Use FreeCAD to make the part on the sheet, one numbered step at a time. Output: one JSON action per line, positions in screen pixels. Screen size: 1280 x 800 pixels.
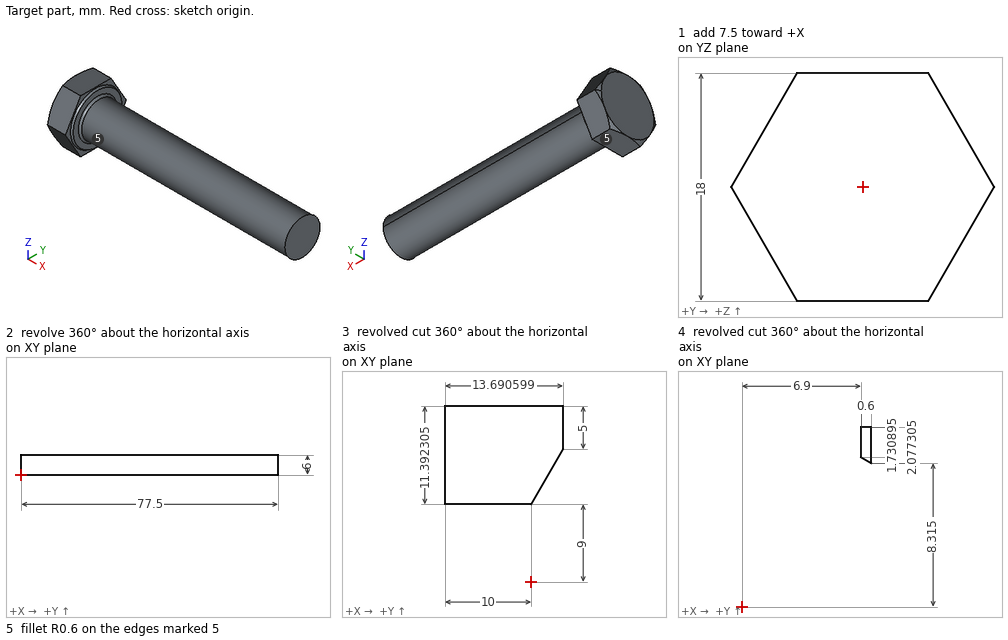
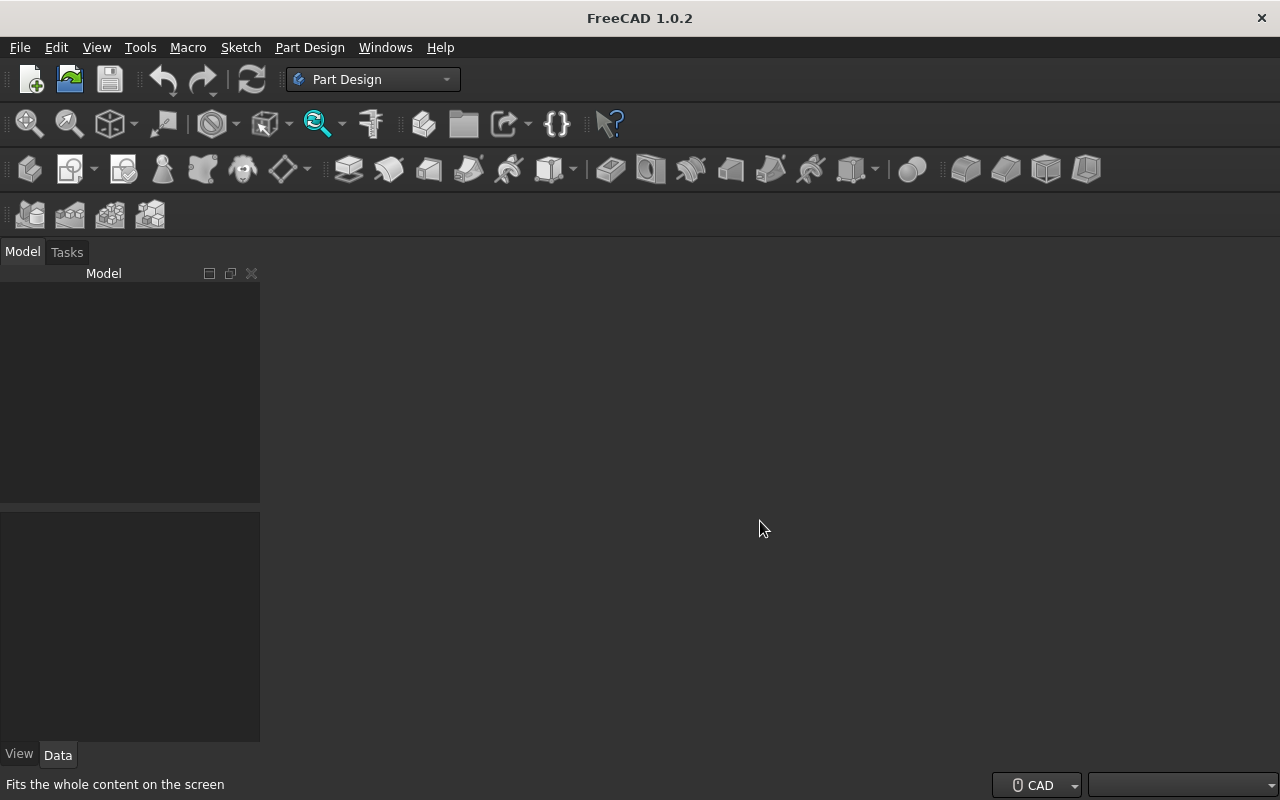
{"action": "left_click", "coordinate": [30, 80]}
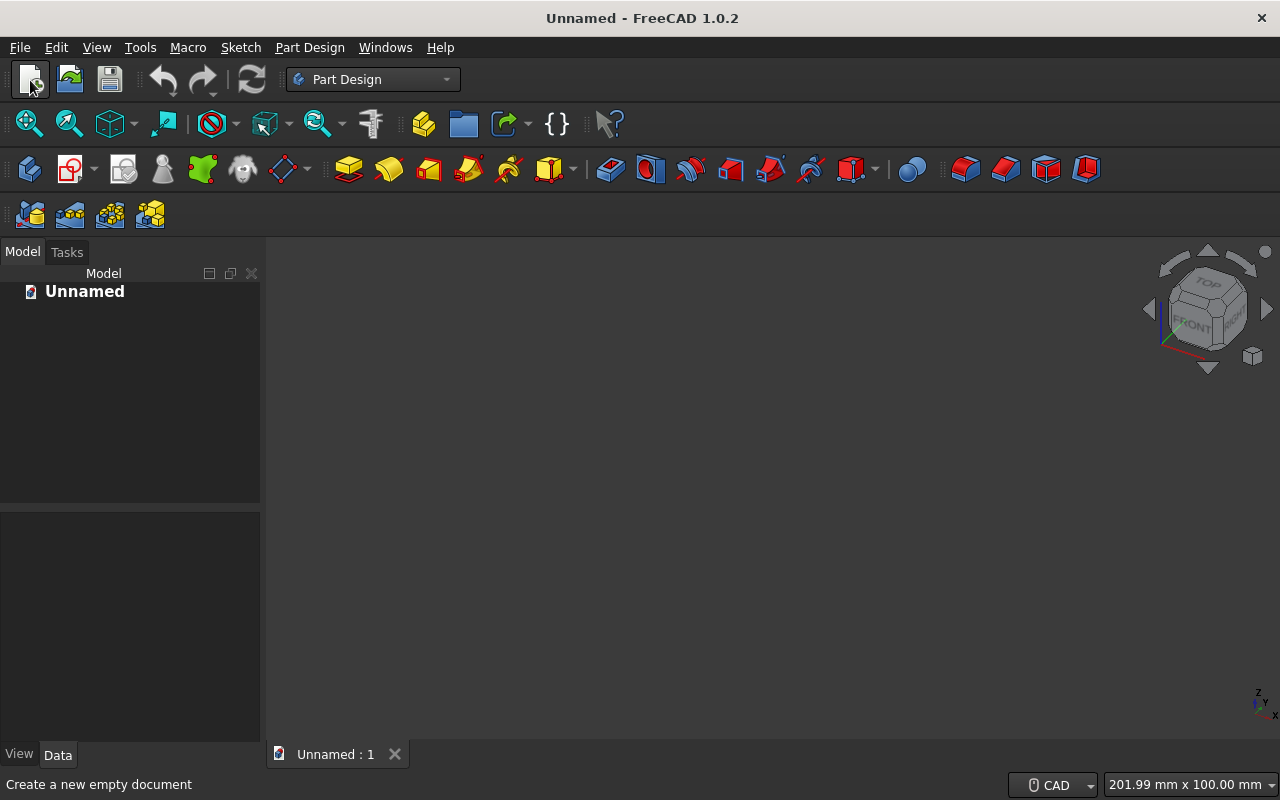
{"action": "left_click", "coordinate": [70, 170]}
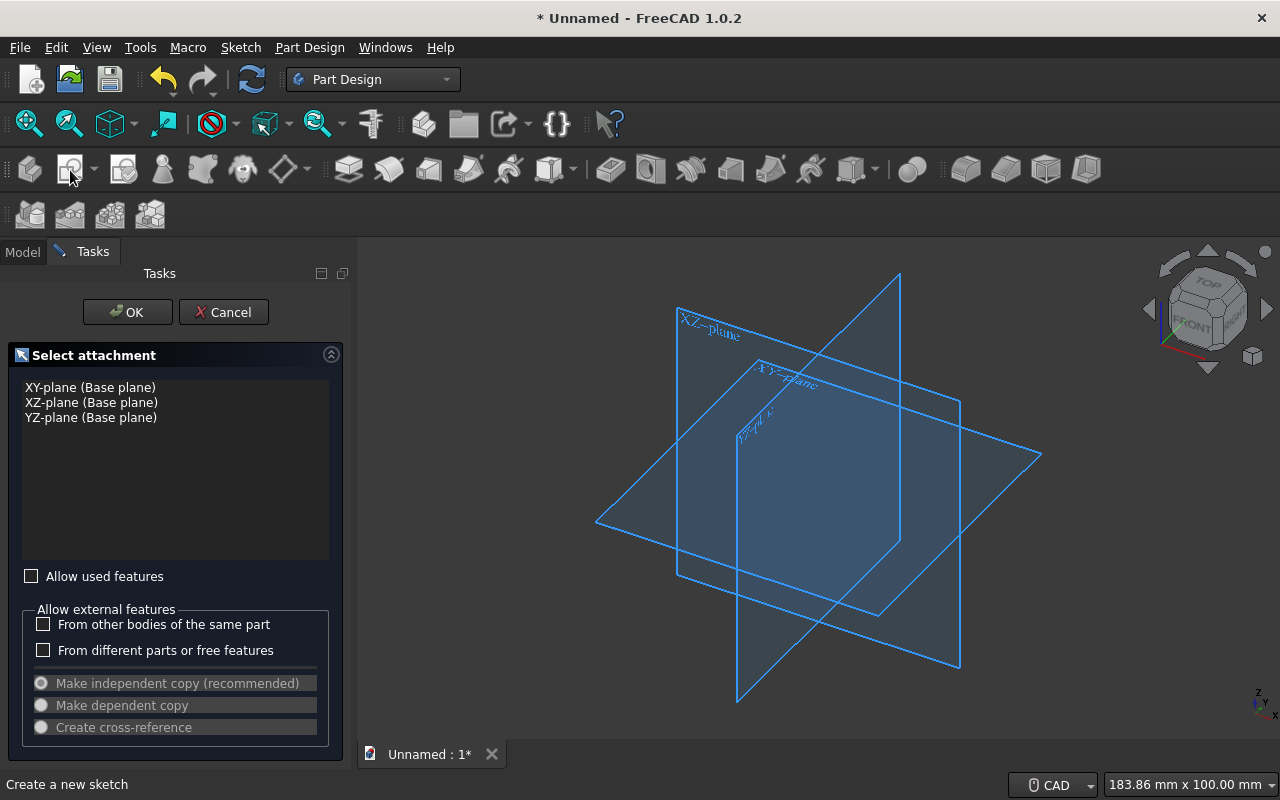
{"action": "left_click", "coordinate": [82, 418]}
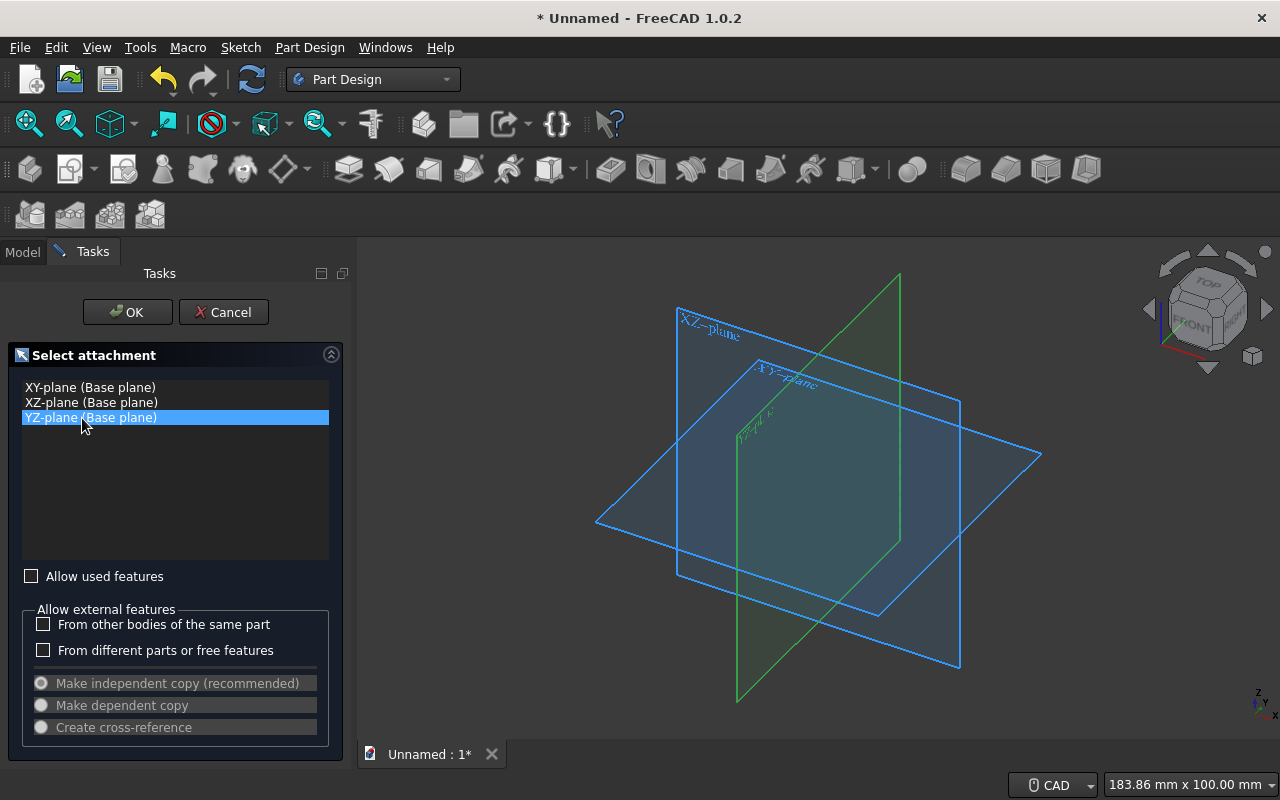
{"action": "left_click", "coordinate": [128, 312]}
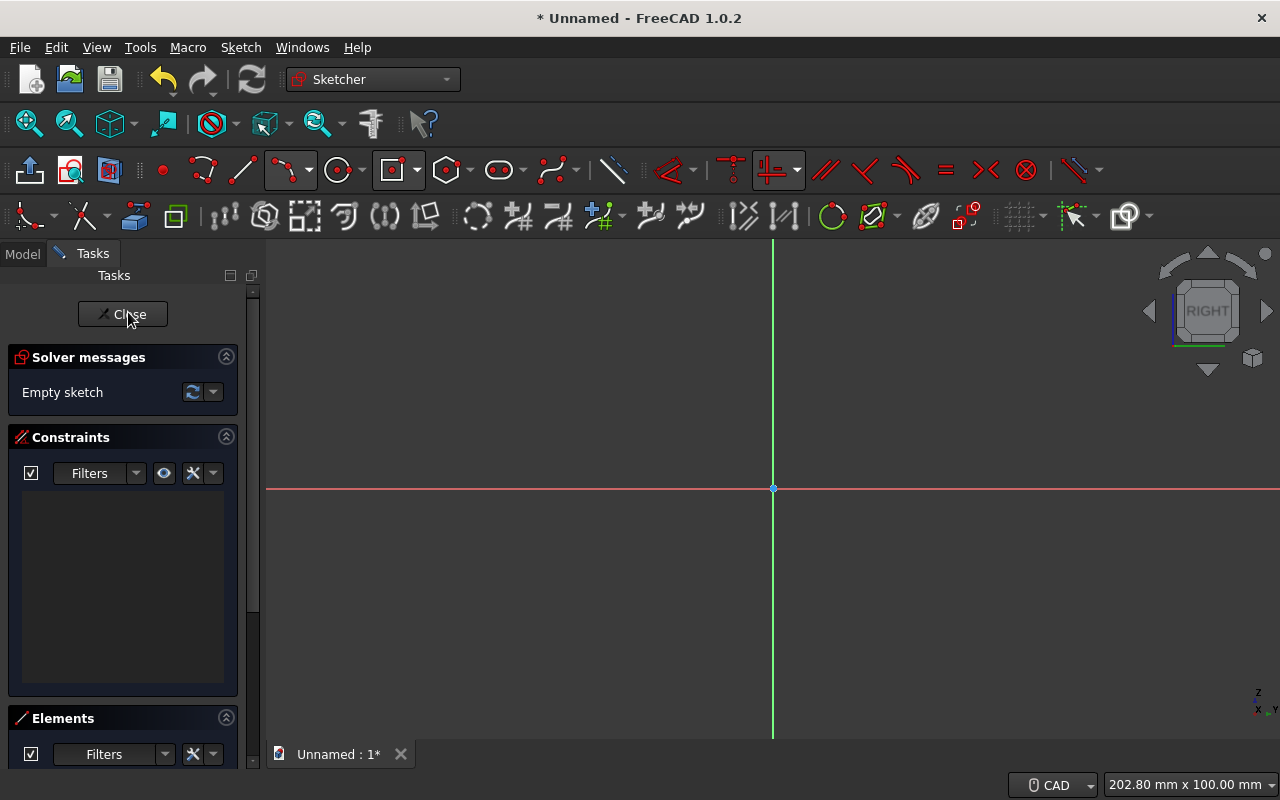
{"action": "scroll", "coordinate": [803, 489], "scroll_direction": "up", "scroll_amount": 6}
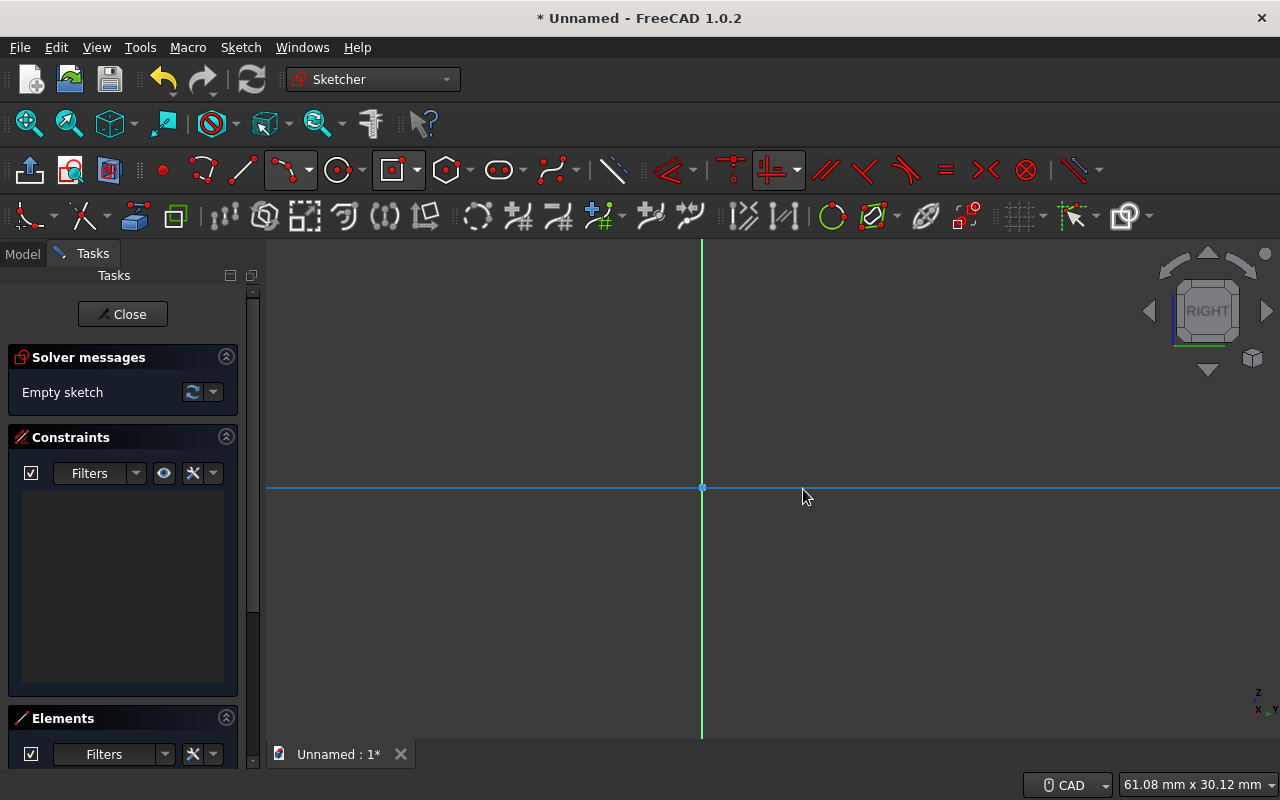
{"action": "left_click", "coordinate": [446, 170]}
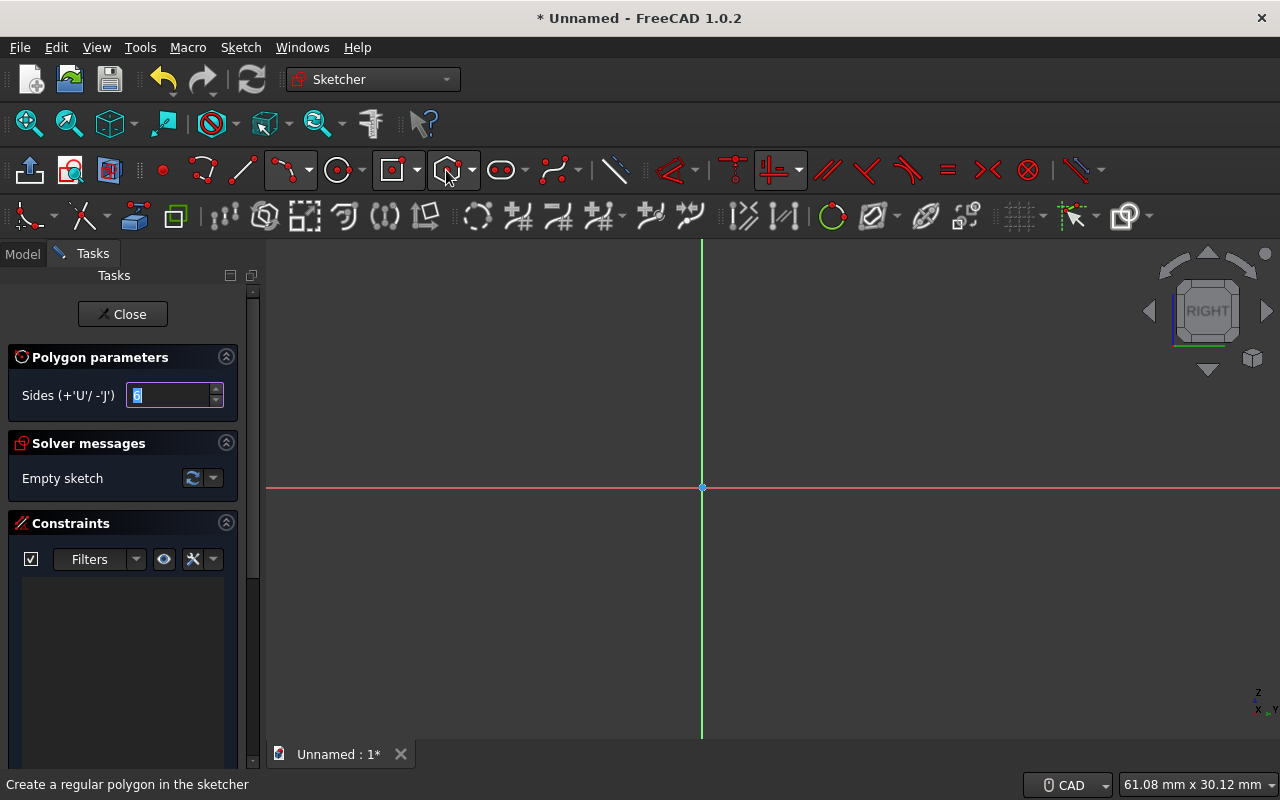
{"action": "left_click", "coordinate": [702, 488]}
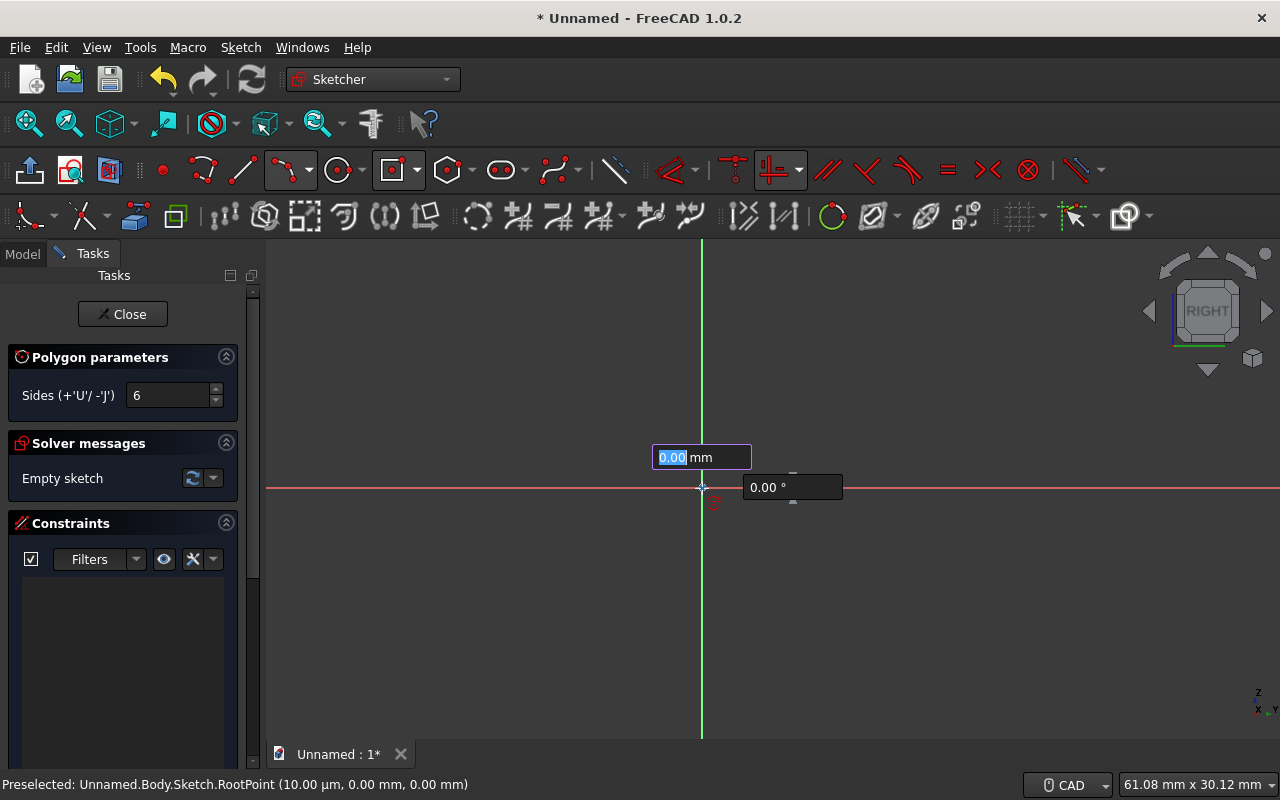
{"action": "left_click", "coordinate": [875, 488]}
{"action": "key", "text": "Escape"}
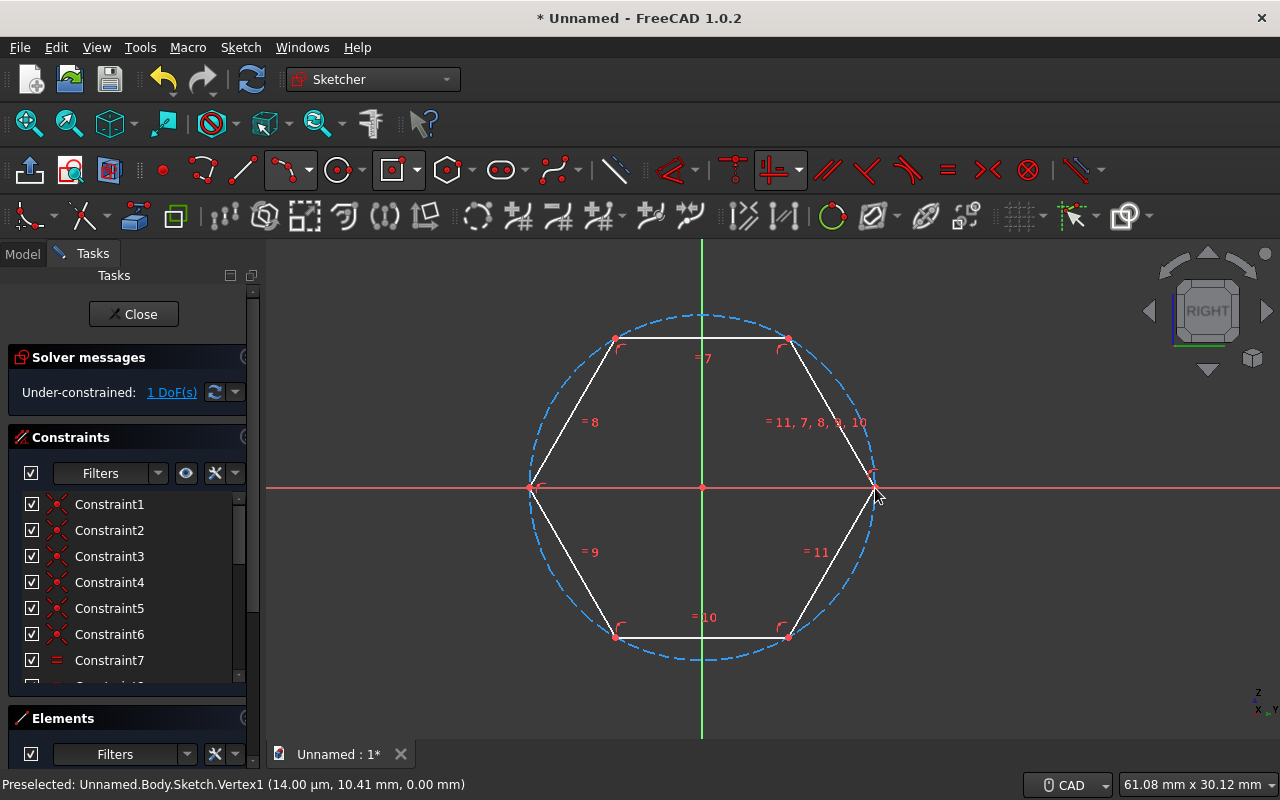
{"action": "left_click", "coordinate": [670, 170]}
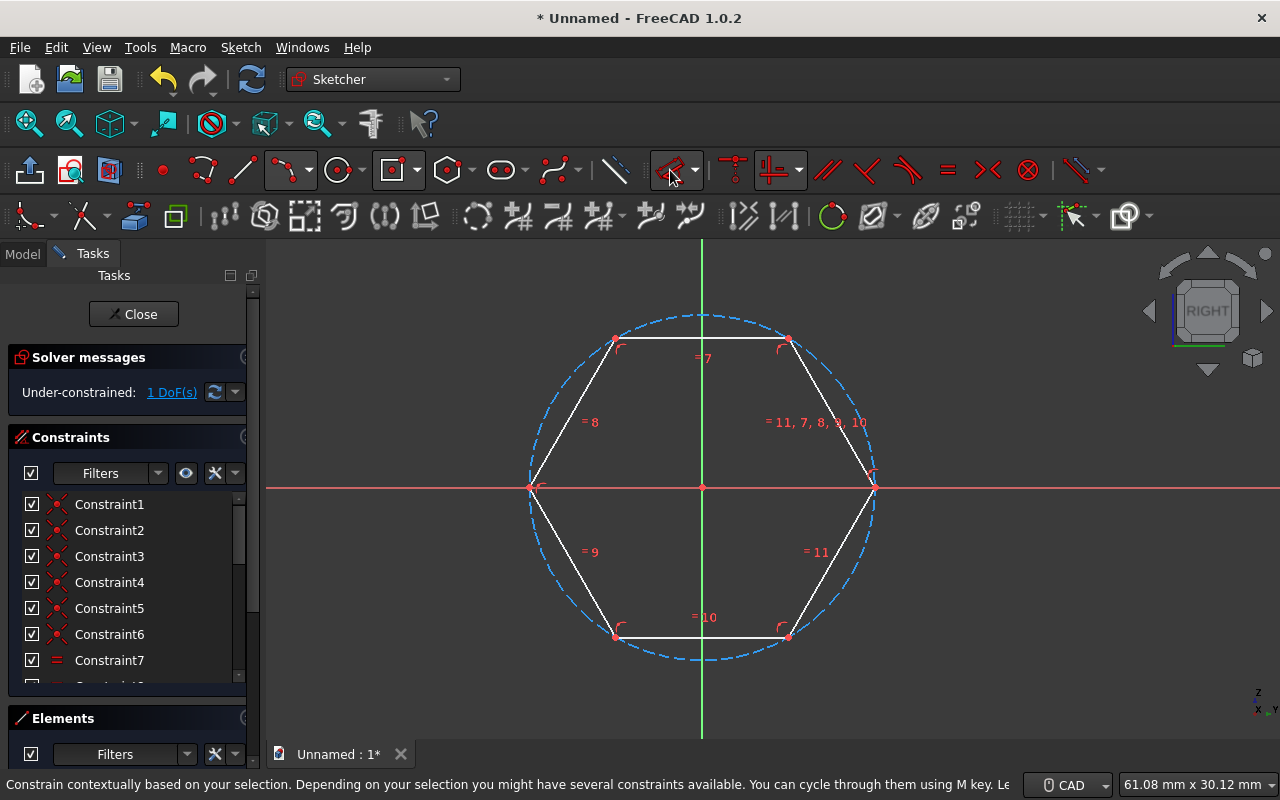
{"action": "left_click", "coordinate": [616, 638]}